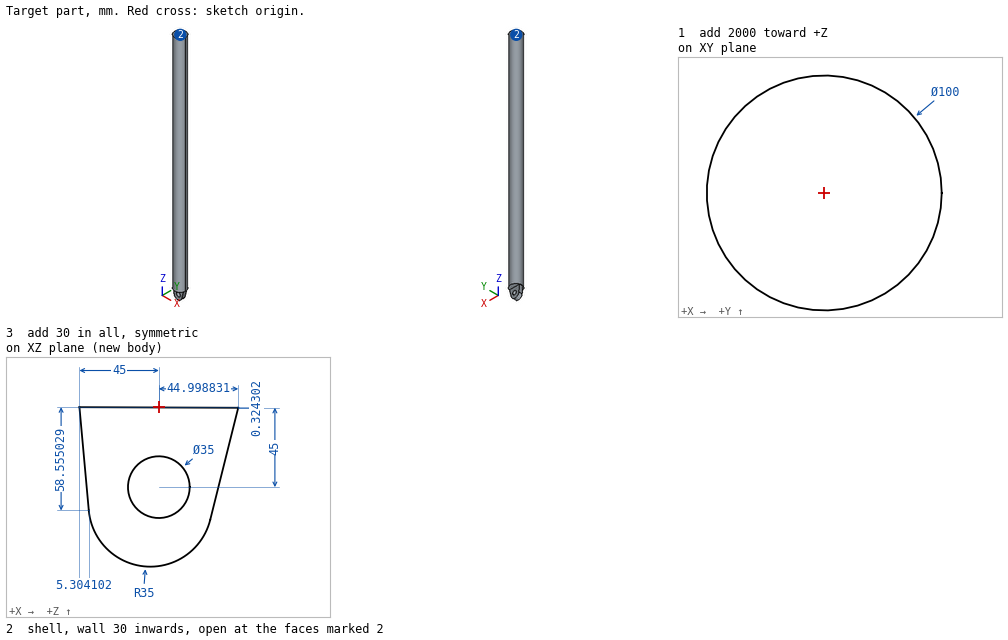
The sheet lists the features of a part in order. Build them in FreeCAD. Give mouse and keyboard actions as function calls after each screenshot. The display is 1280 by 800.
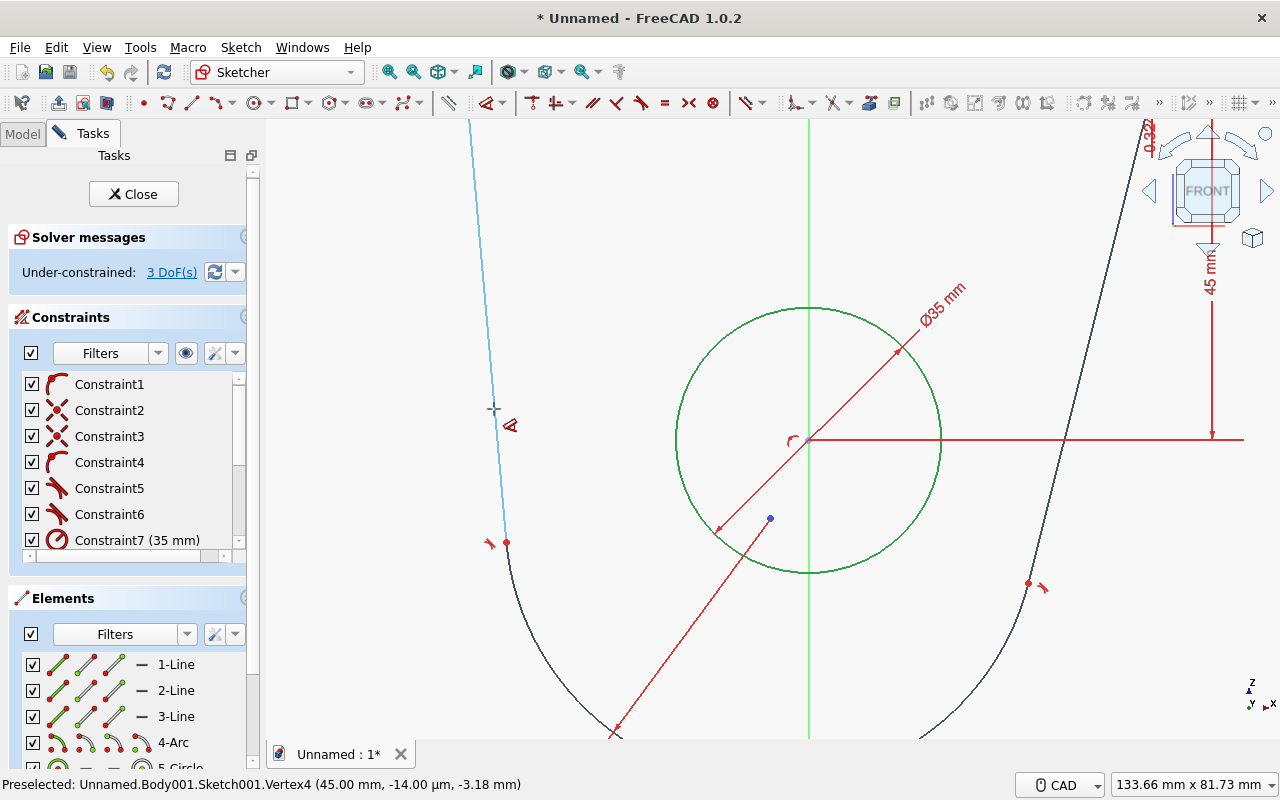
click(495, 408)
click(487, 576)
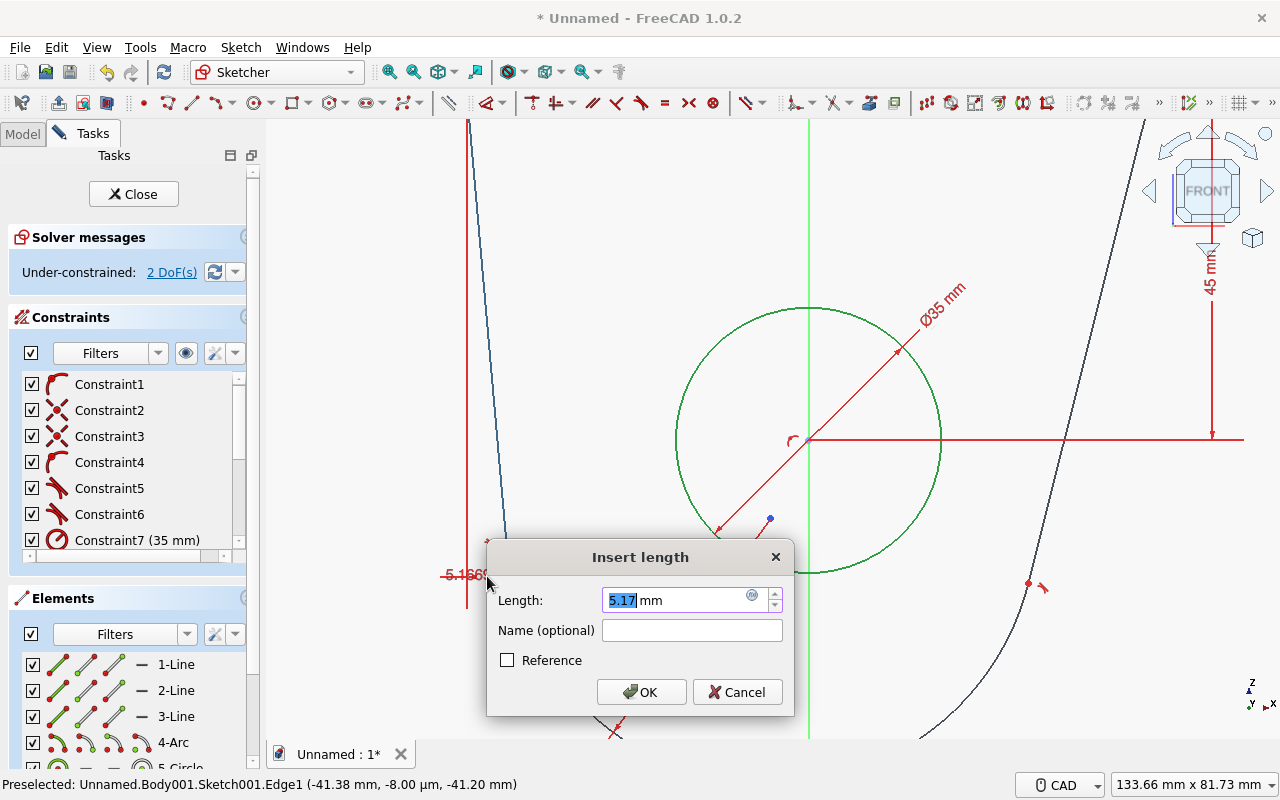
text(5.304102)
key(Return)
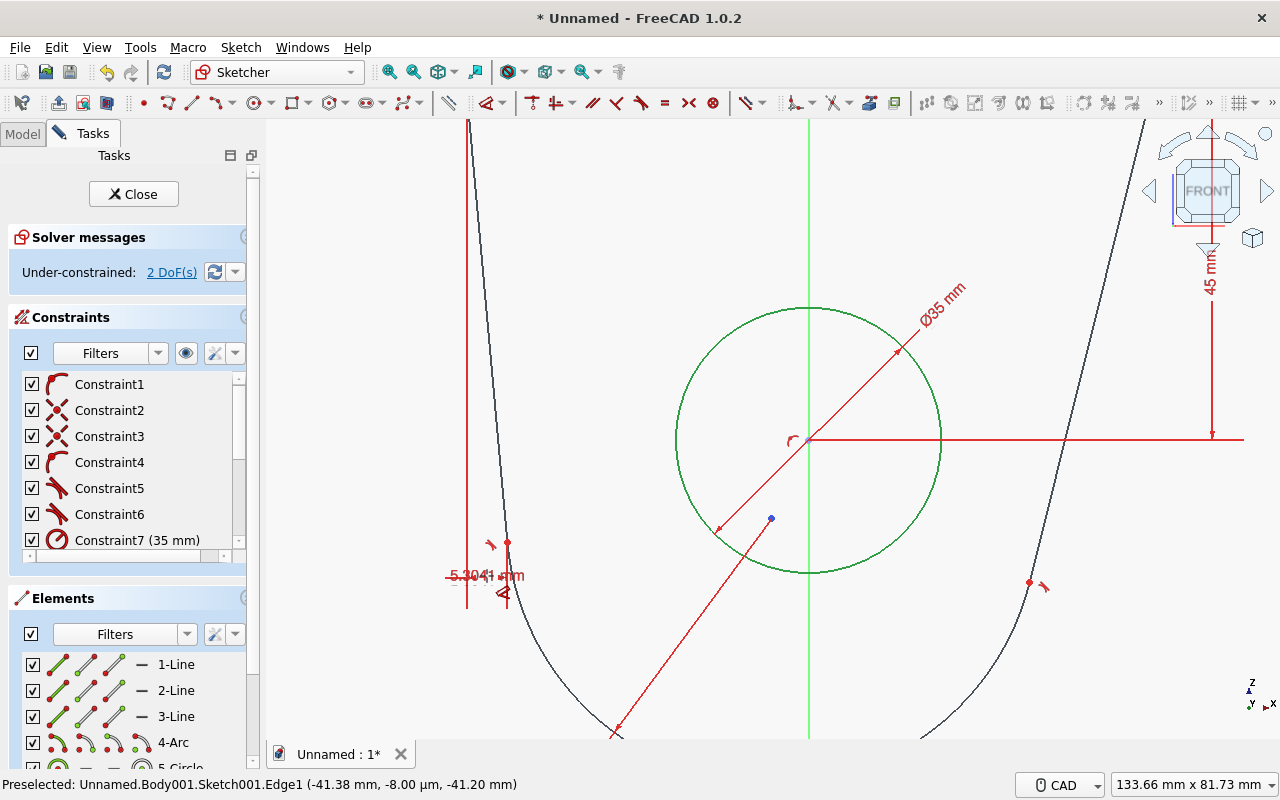
click(507, 543)
click(473, 345)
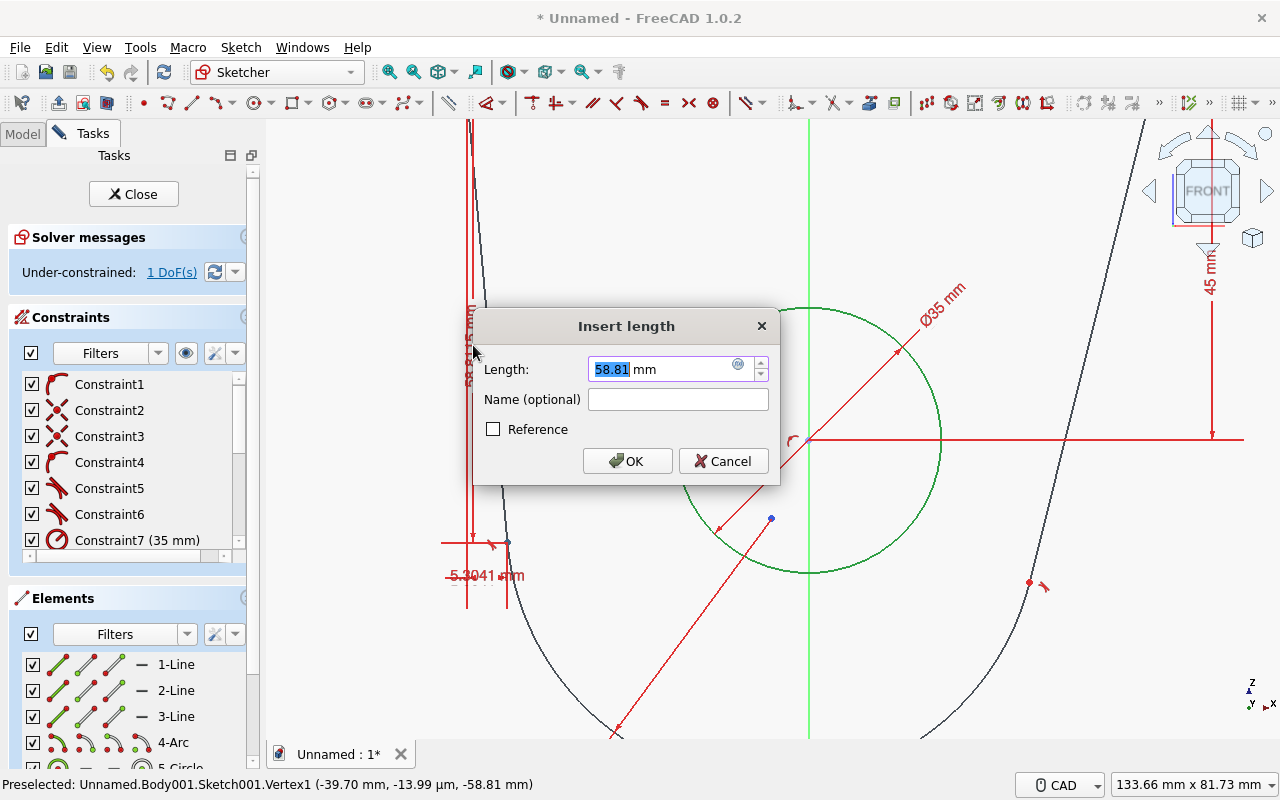
text(58.555029)
key(Return)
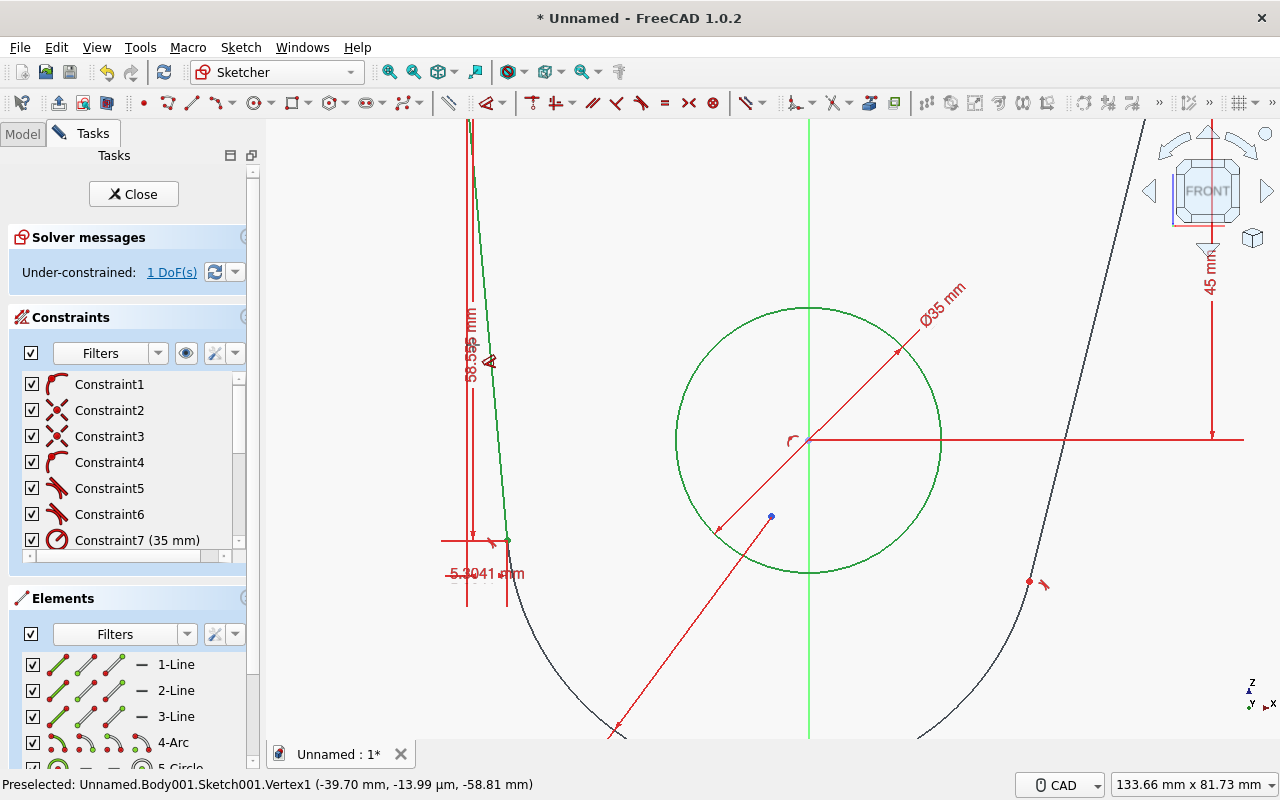
scroll(578, 417, down, 3)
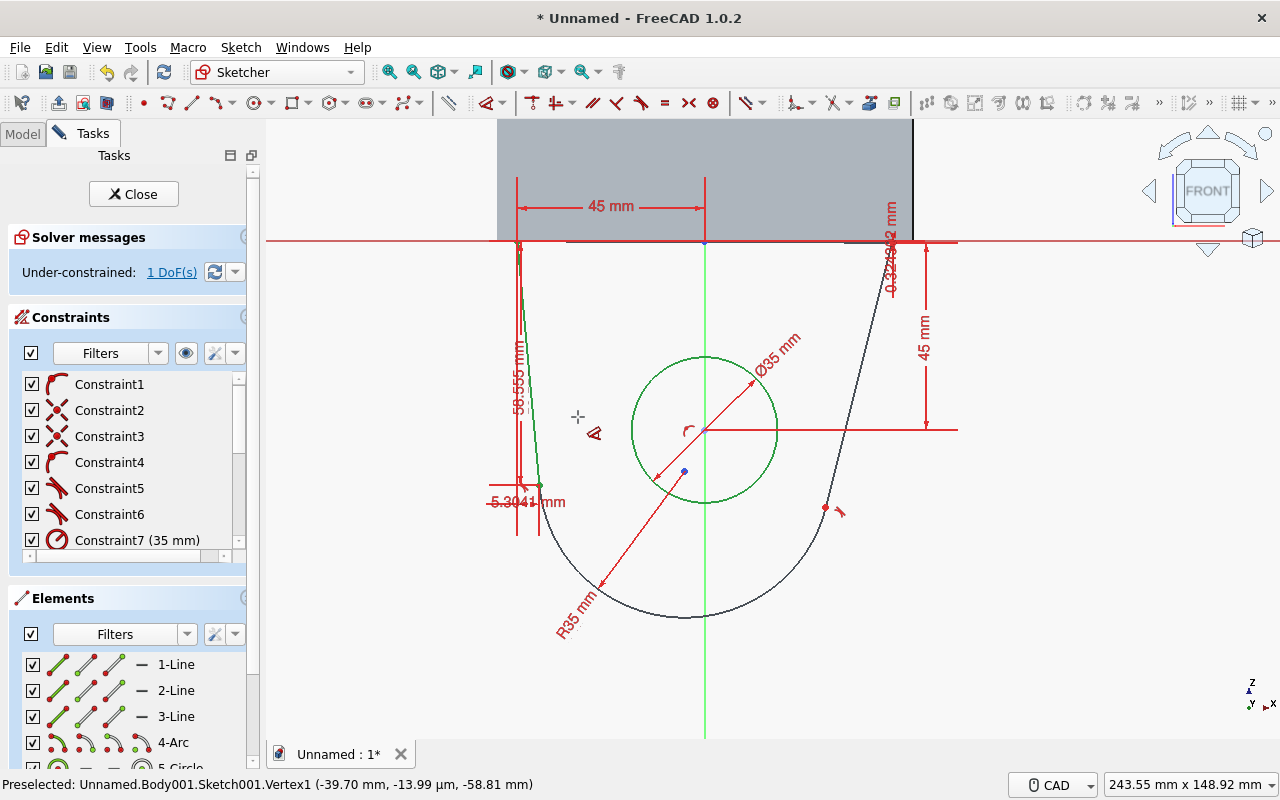
click(892, 243)
click(798, 207)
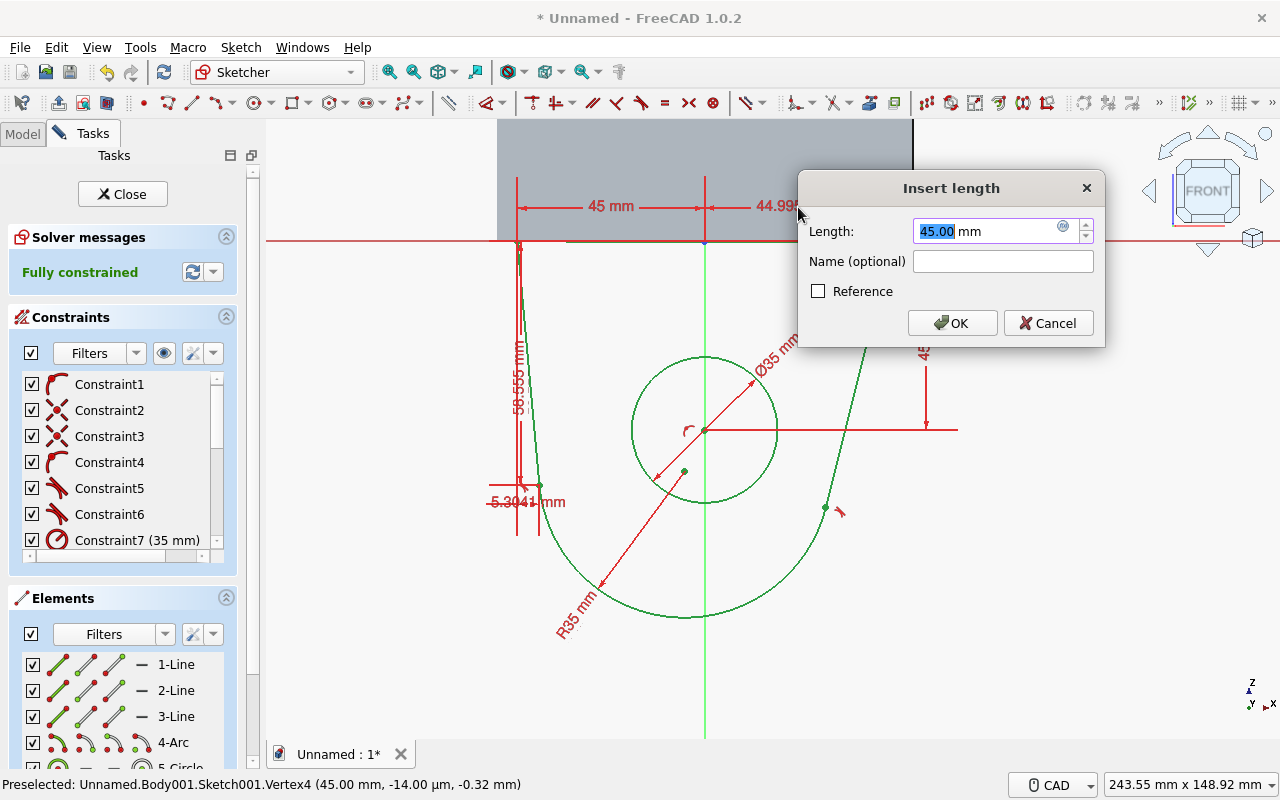
text(44.998831)
key(Return)
key(Escape)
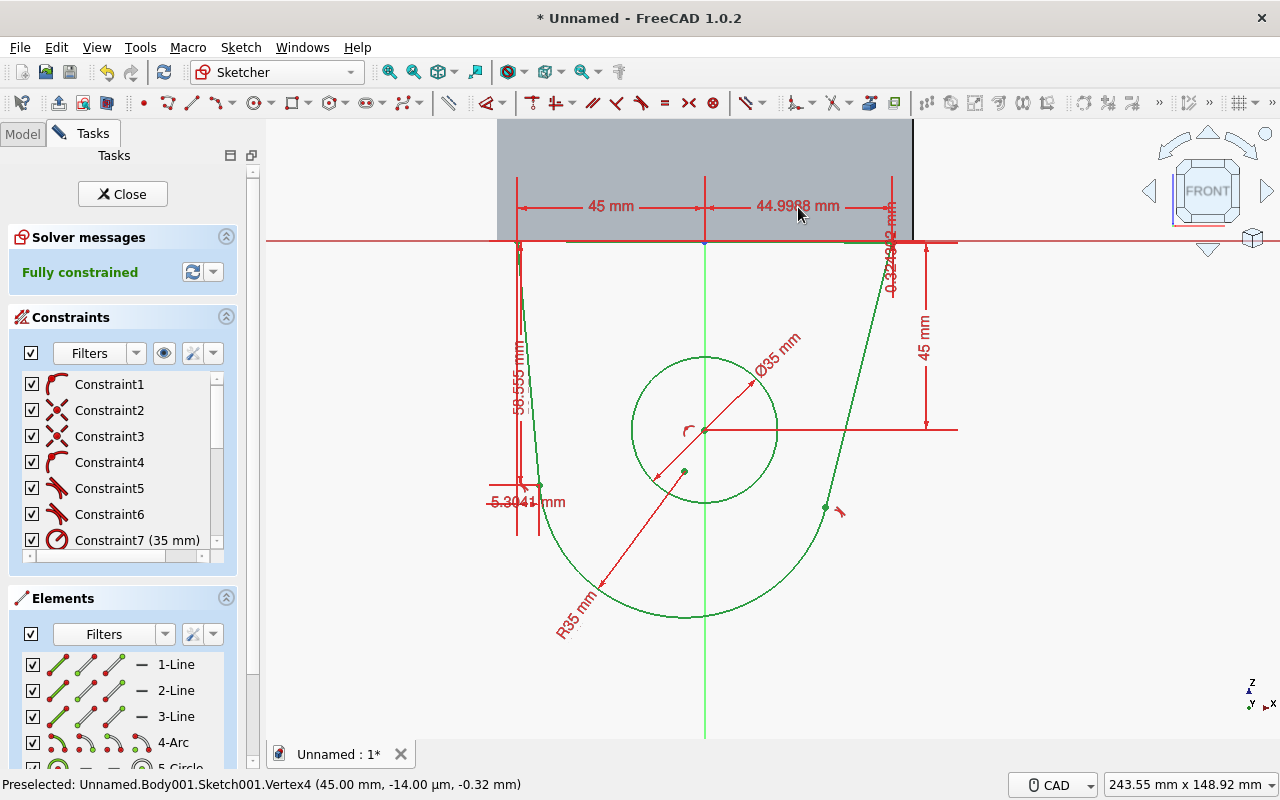
click(123, 194)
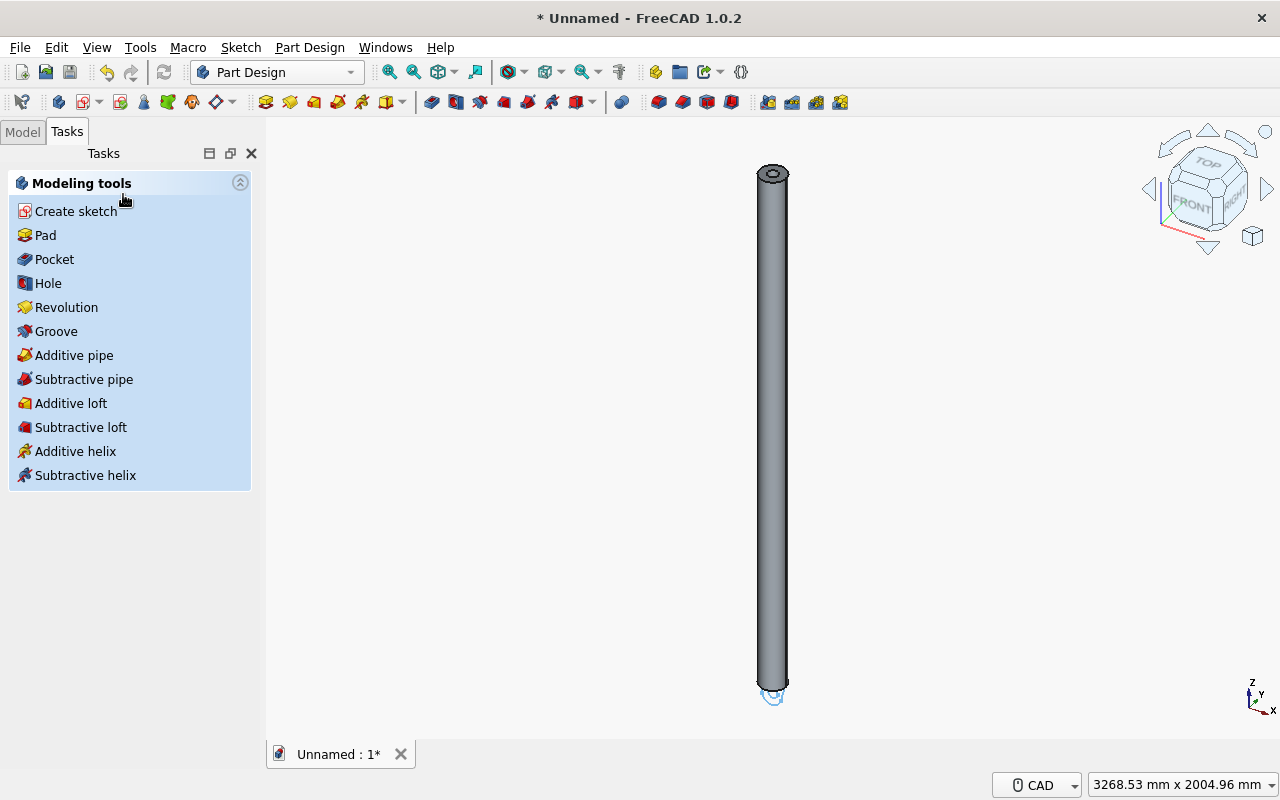
click(266, 102)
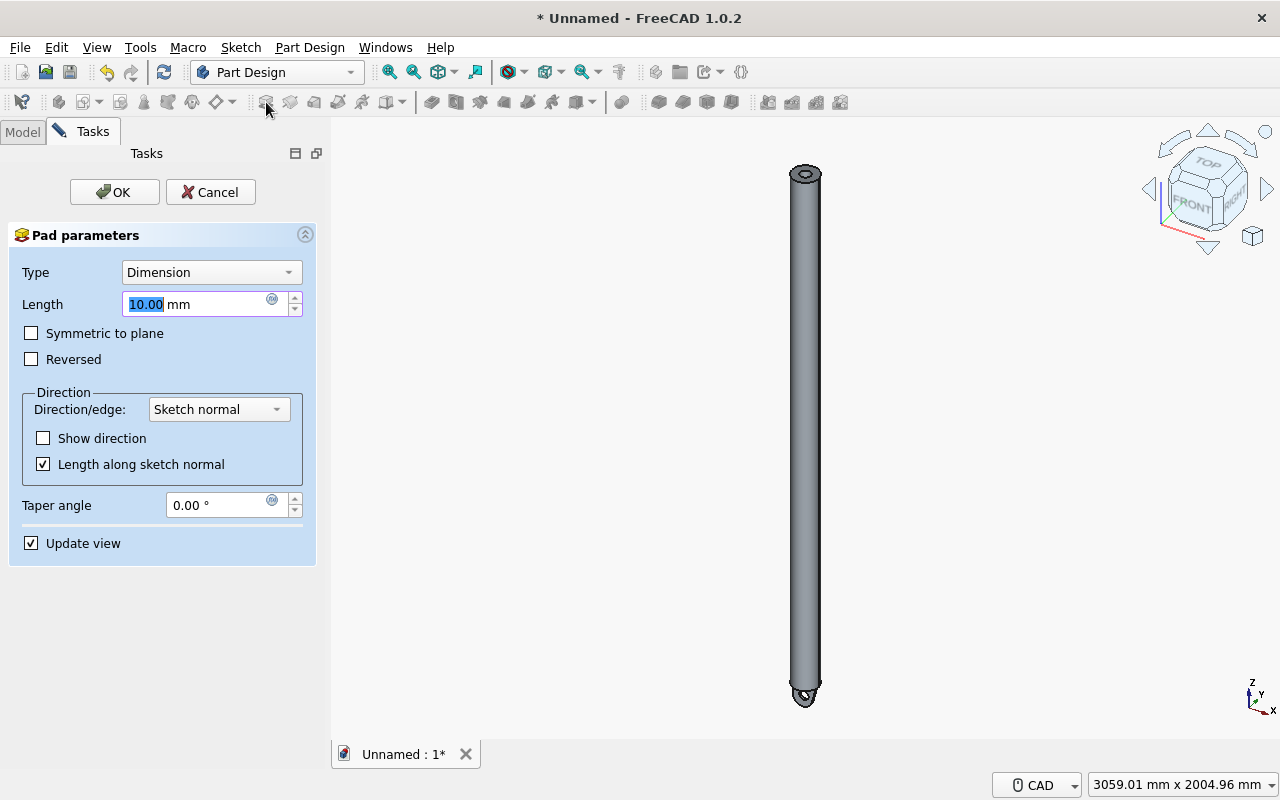
text(30)
key(Tab)